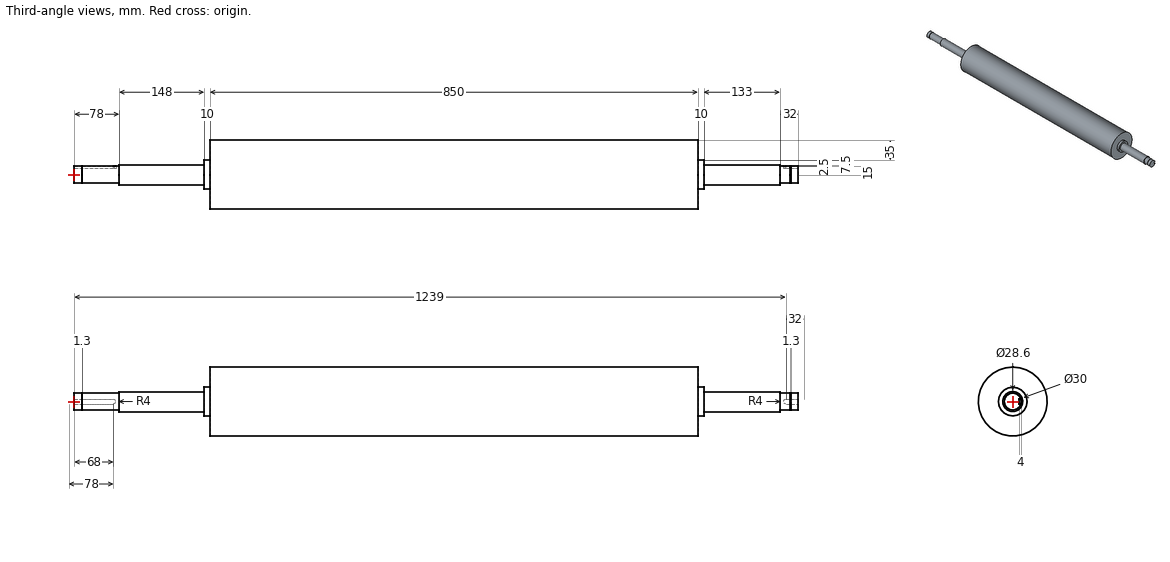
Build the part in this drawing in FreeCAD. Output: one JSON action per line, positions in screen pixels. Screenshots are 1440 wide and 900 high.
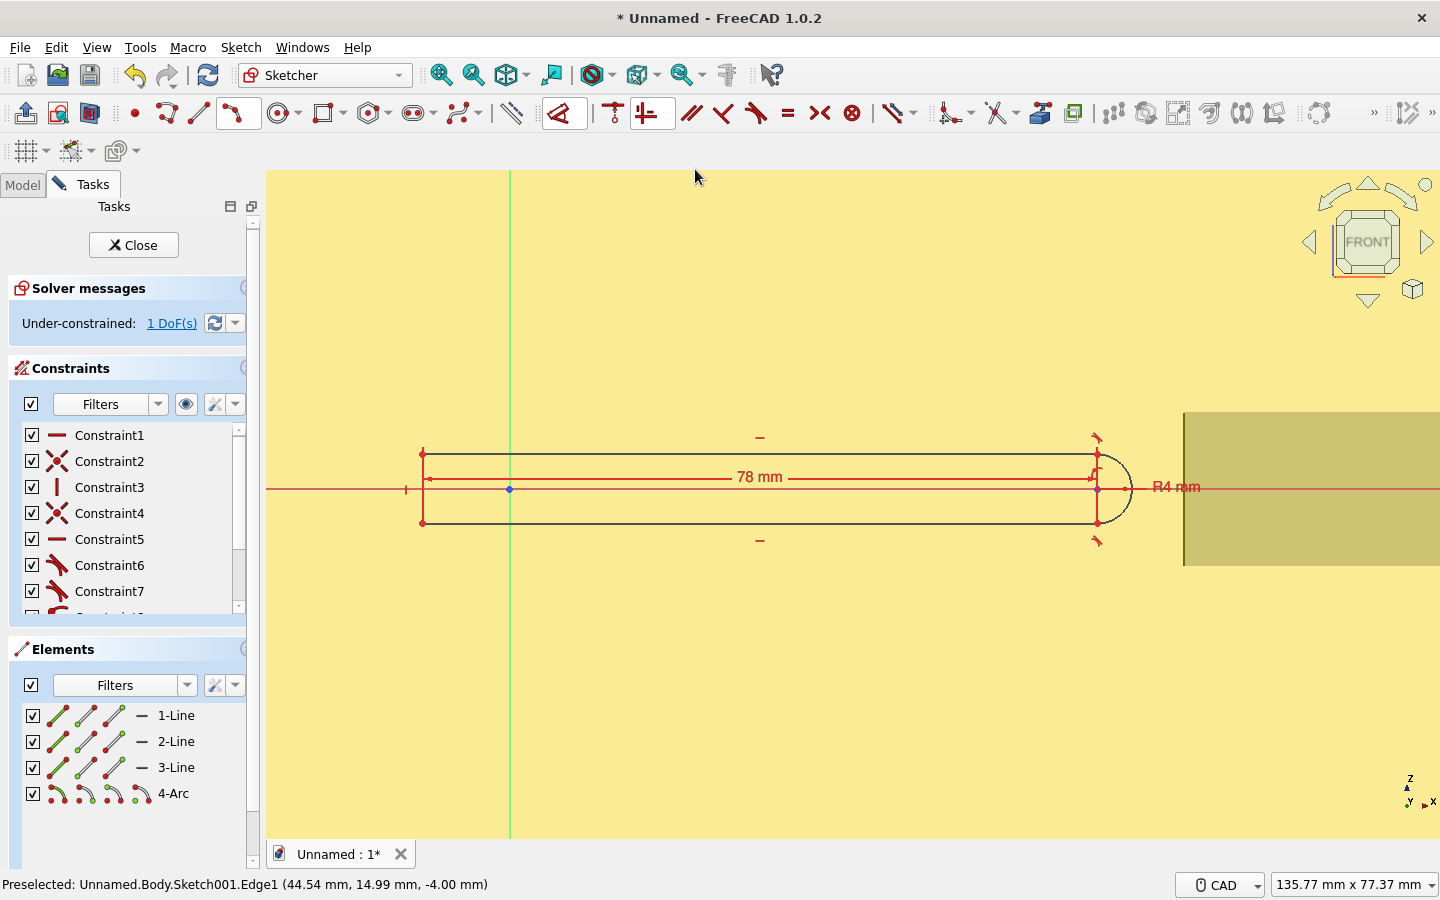
{"action": "left_click", "coordinate": [1097, 524]}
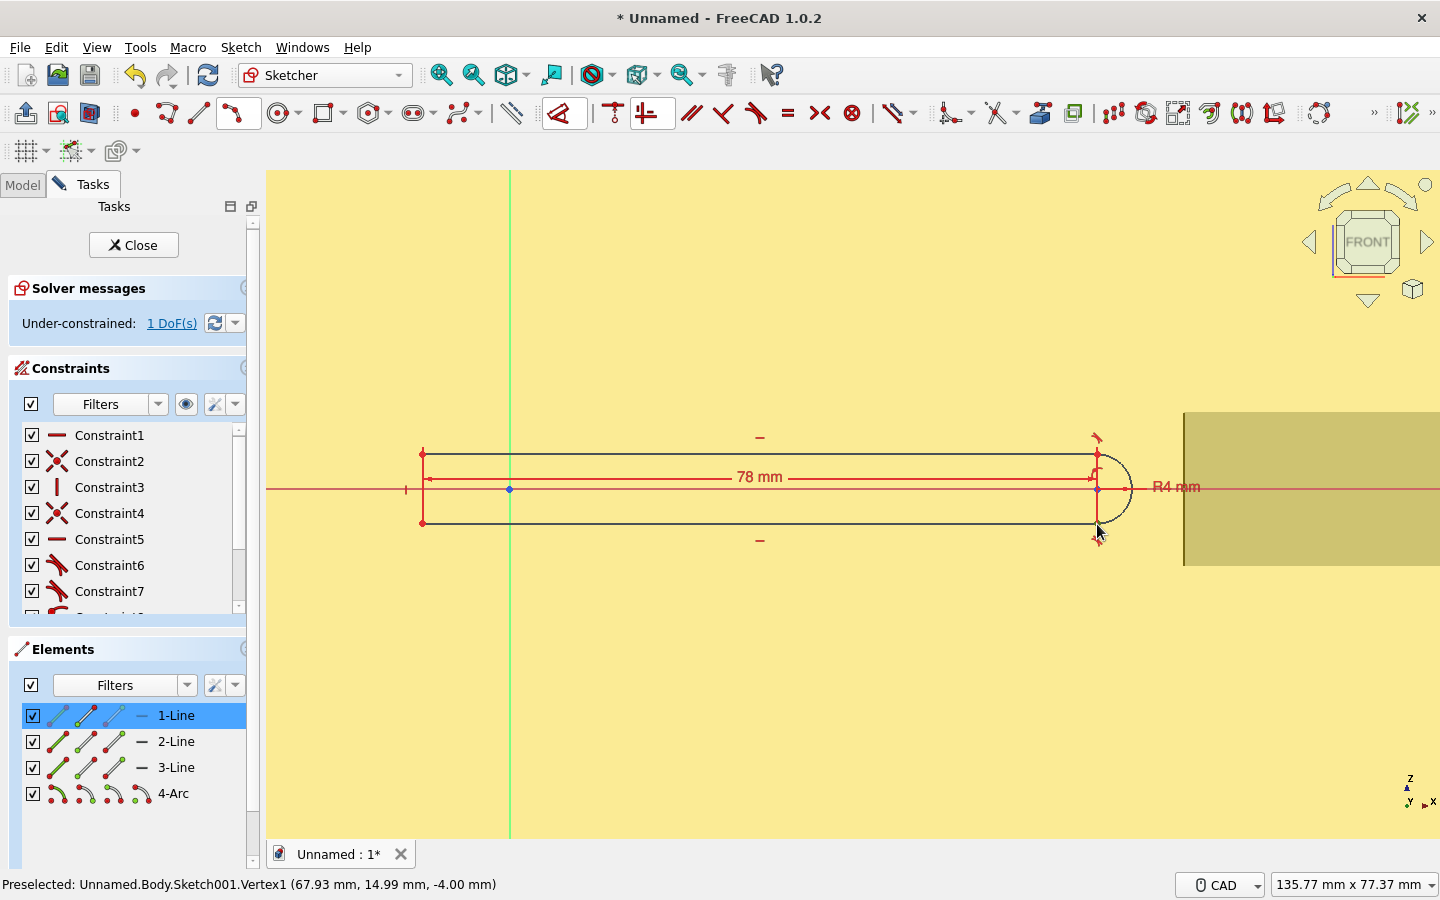
{"action": "key", "text": "l"}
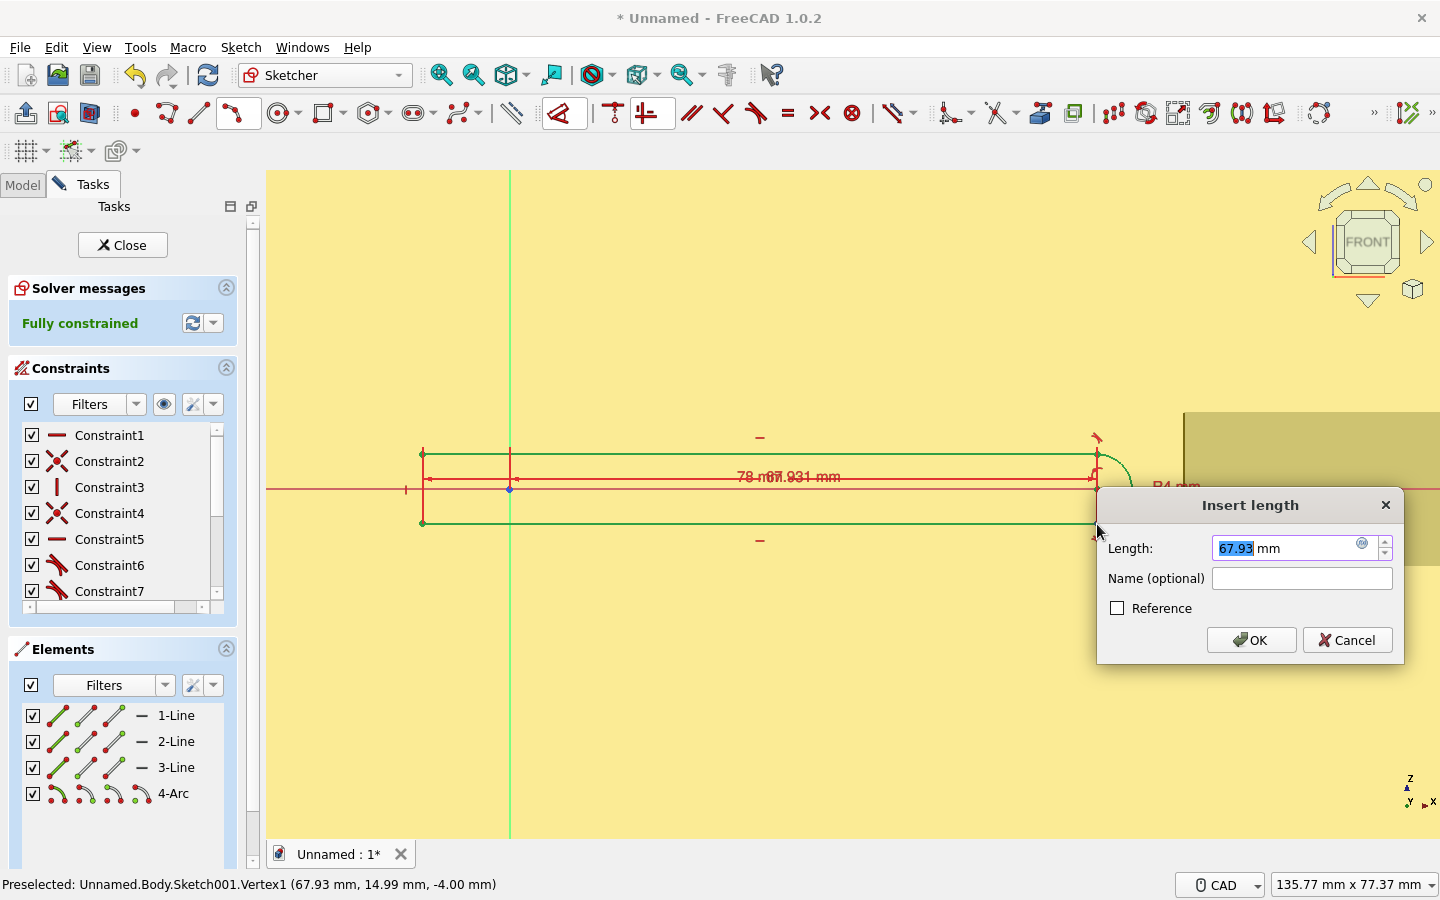
{"action": "type", "text": "68"}
{"action": "key", "text": "Return"}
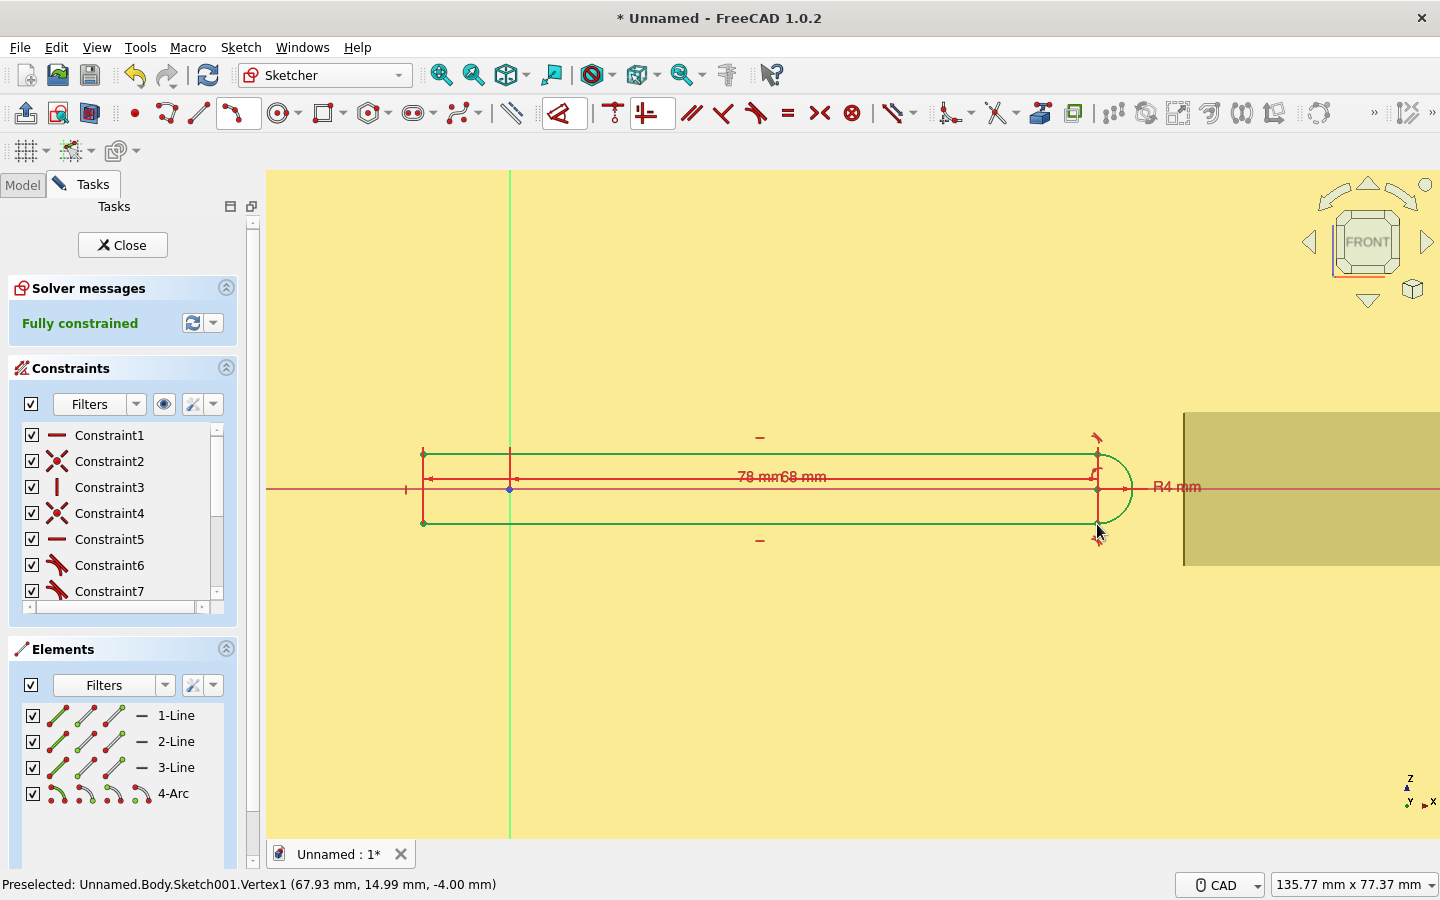
{"action": "left_click", "coordinate": [123, 245]}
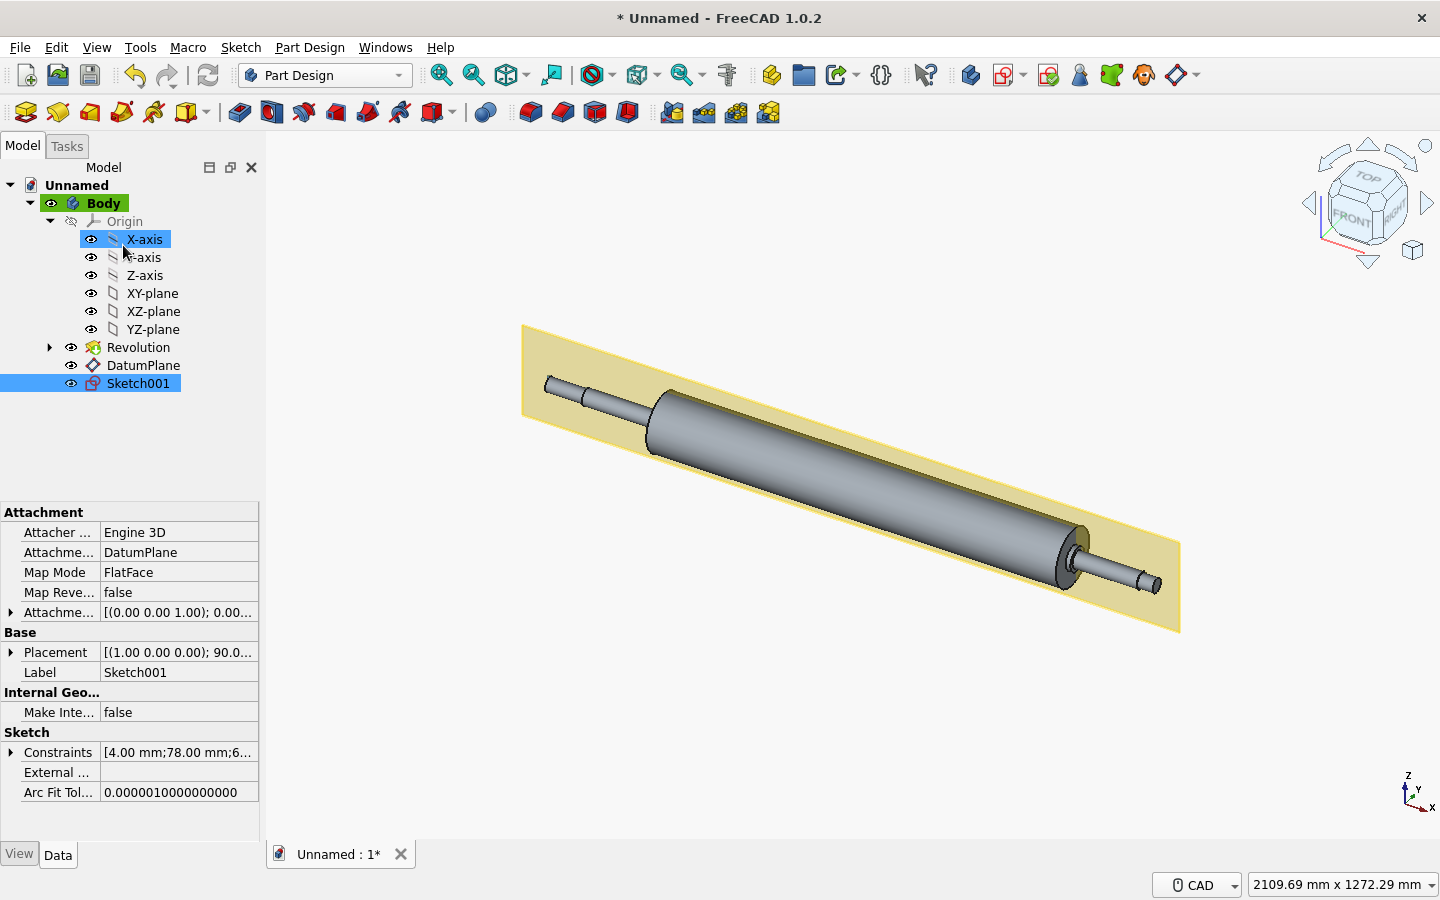
{"action": "left_click", "coordinate": [240, 112]}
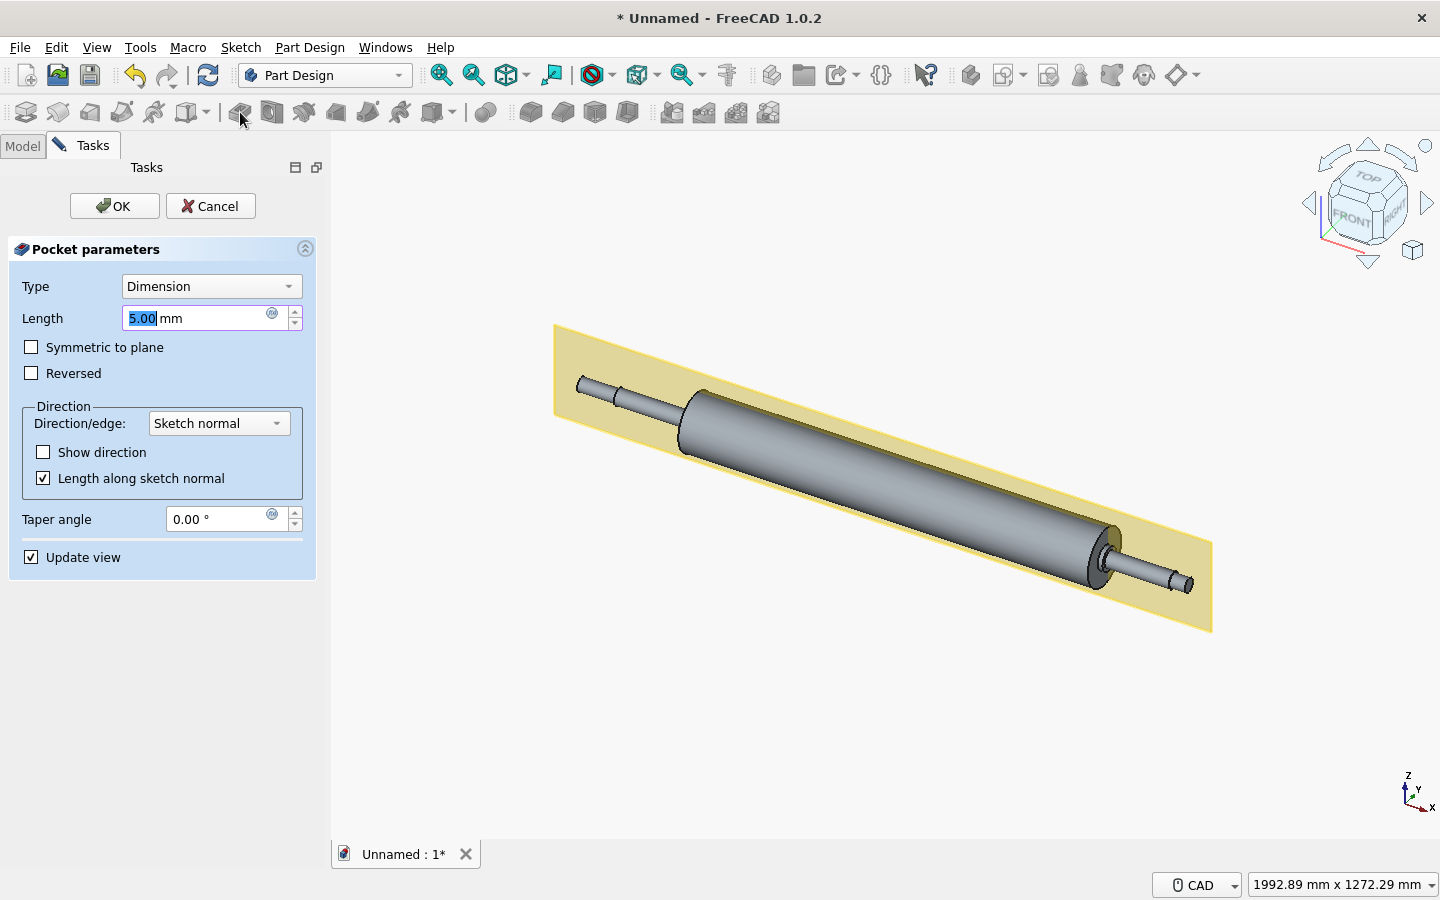
{"action": "type", "text": "4"}
{"action": "key", "text": "Tab"}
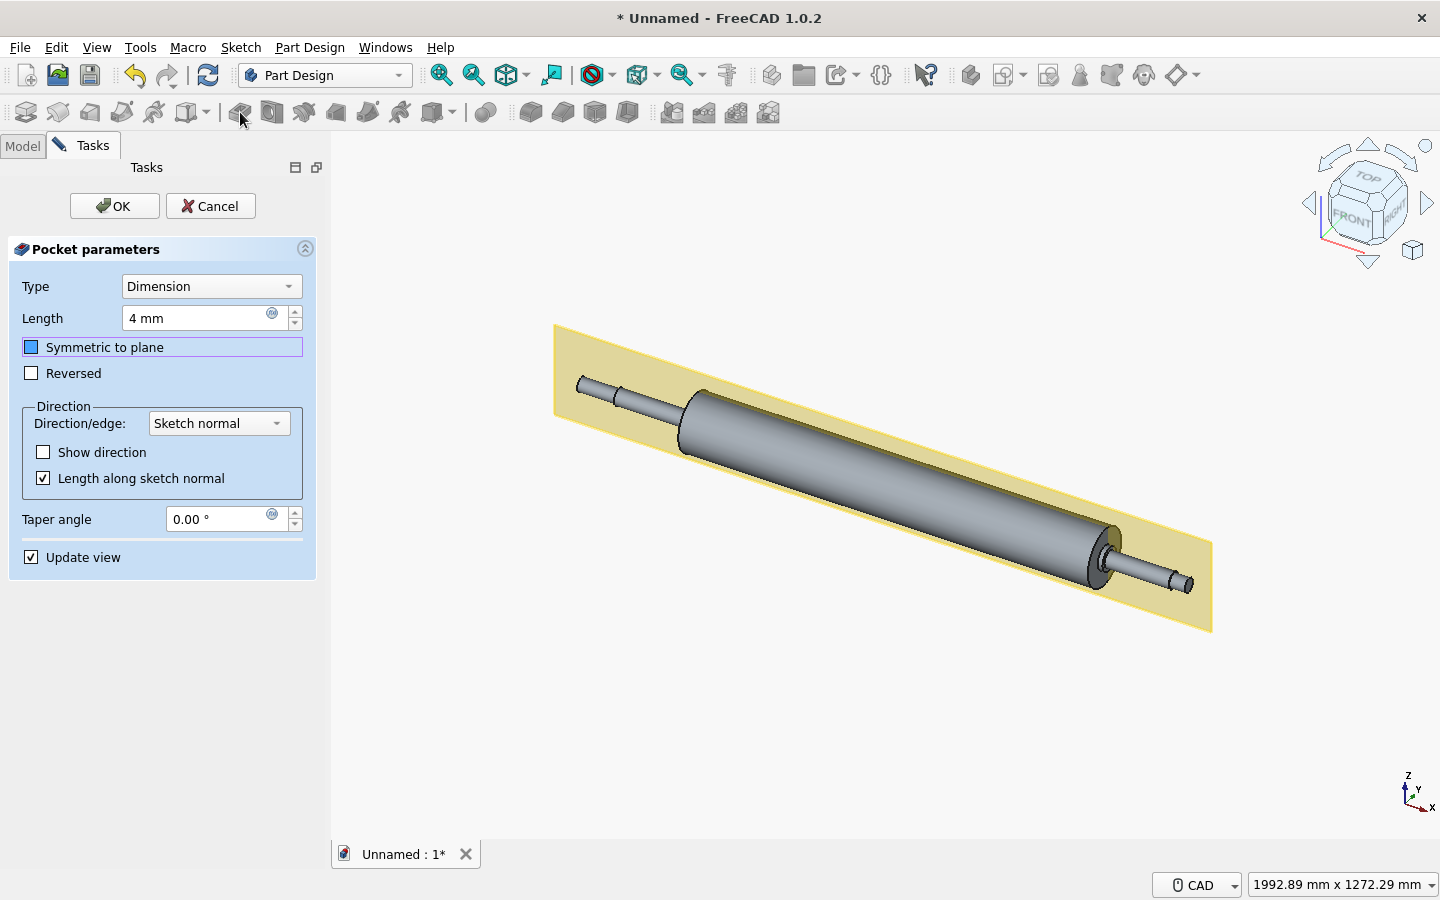
{"action": "left_click", "coordinate": [30, 373]}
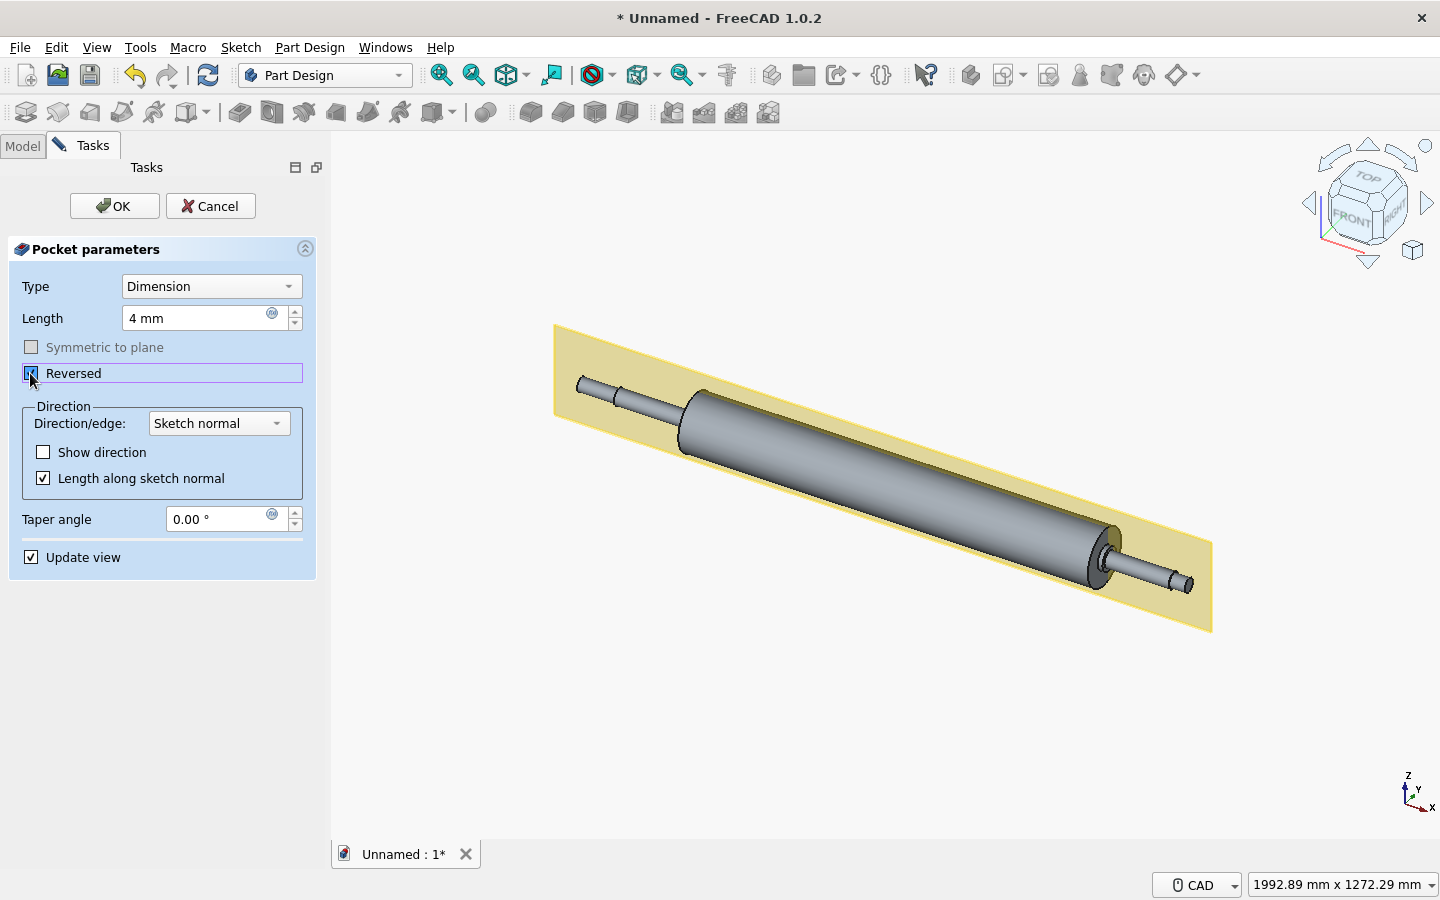
{"action": "left_click", "coordinate": [115, 206]}